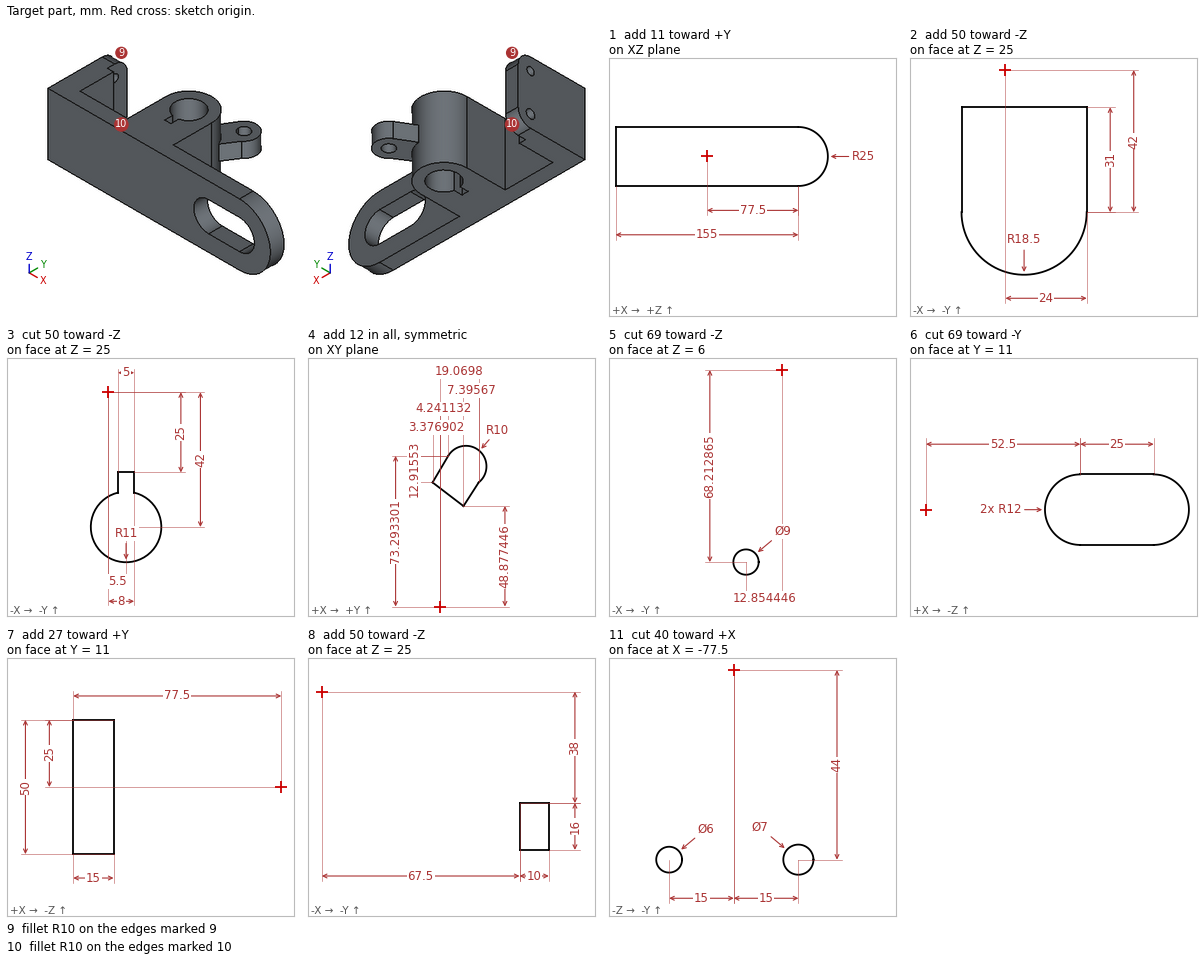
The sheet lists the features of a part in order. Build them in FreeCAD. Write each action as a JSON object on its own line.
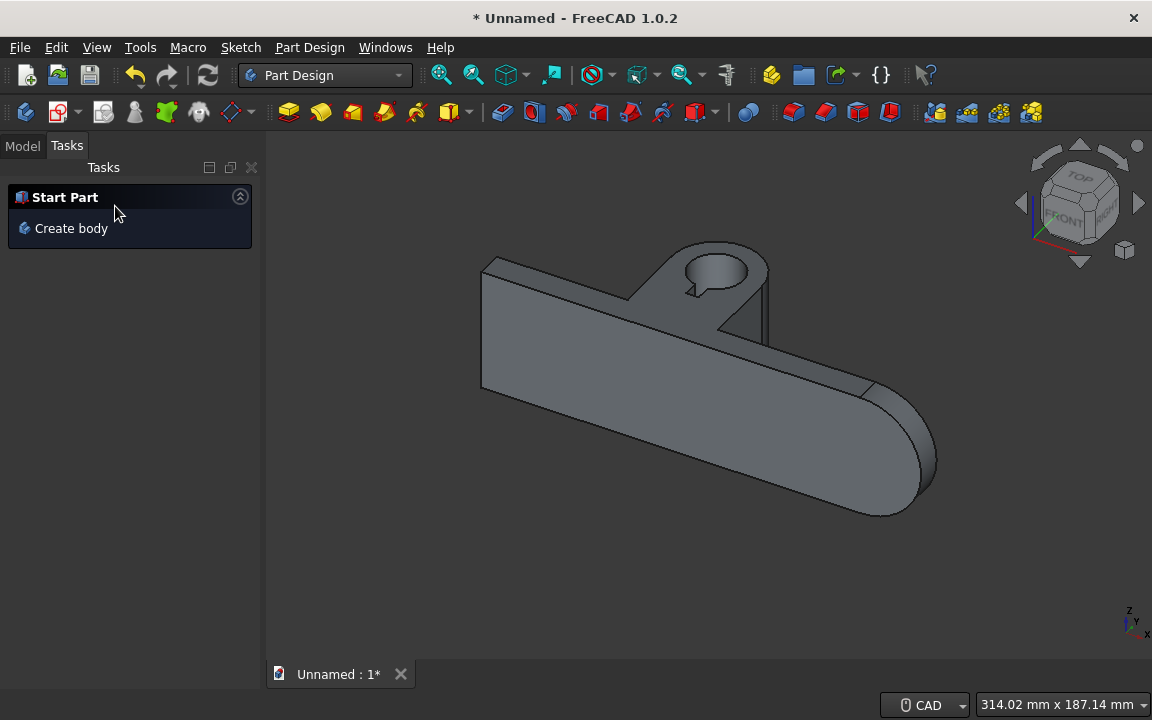
{"action": "left_click", "coordinate": [58, 112]}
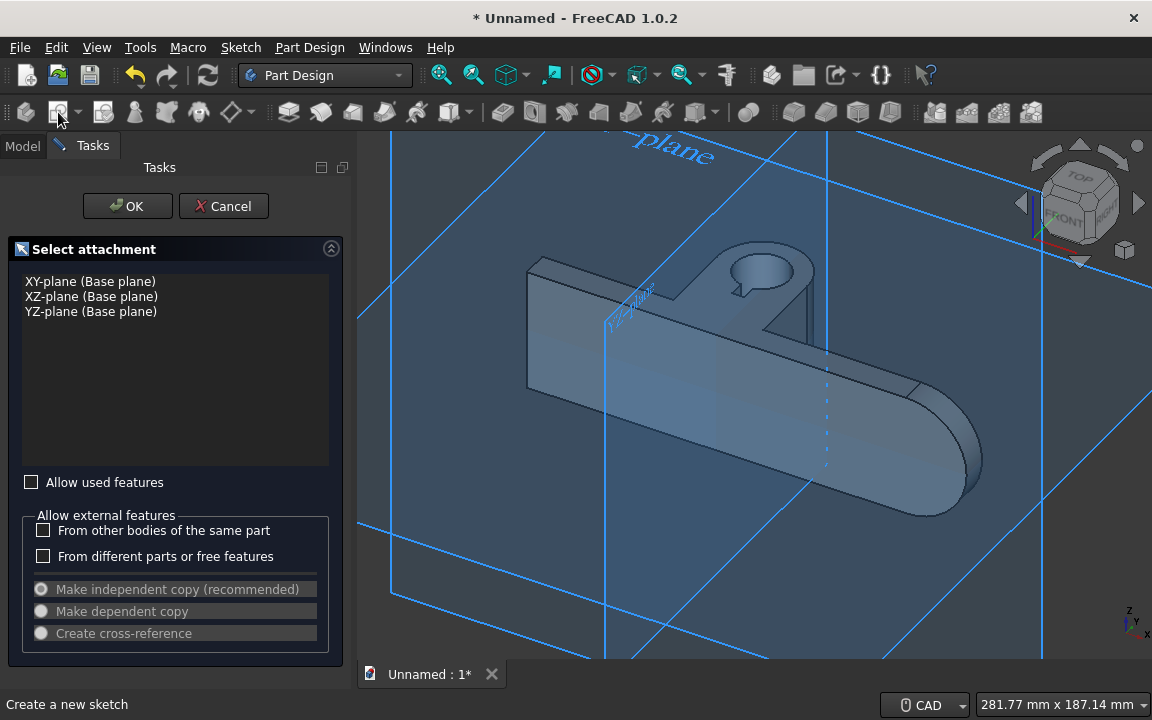
{"action": "left_click", "coordinate": [82, 282]}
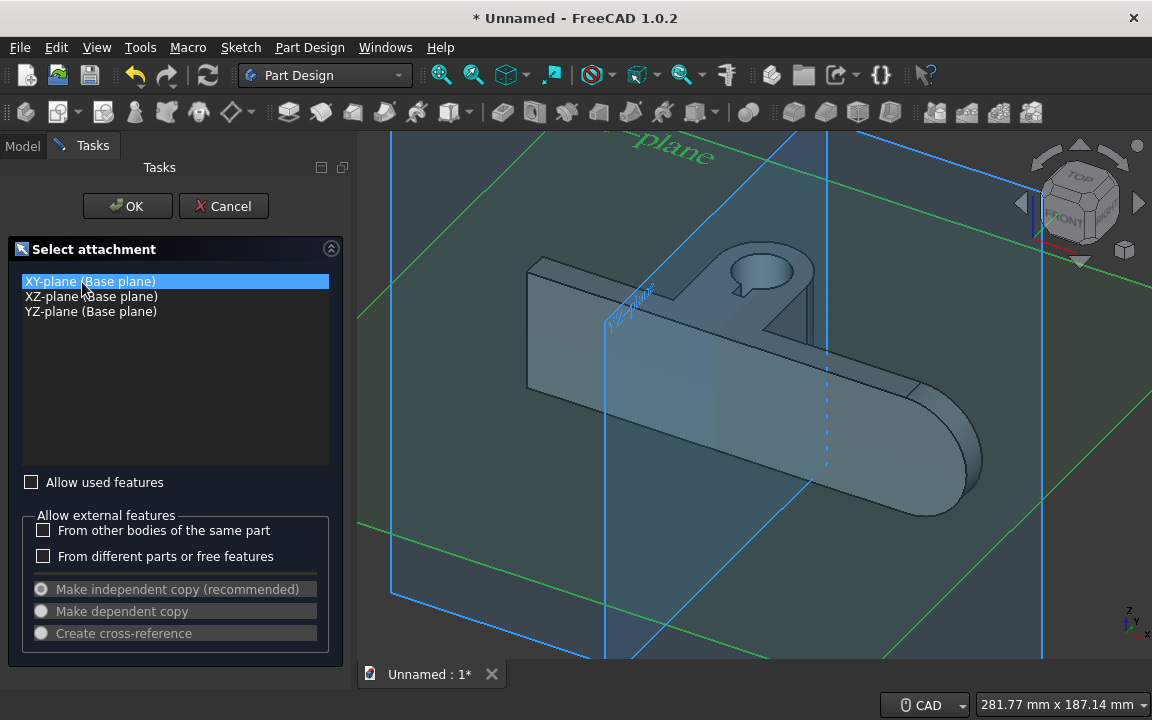
{"action": "left_click", "coordinate": [128, 206]}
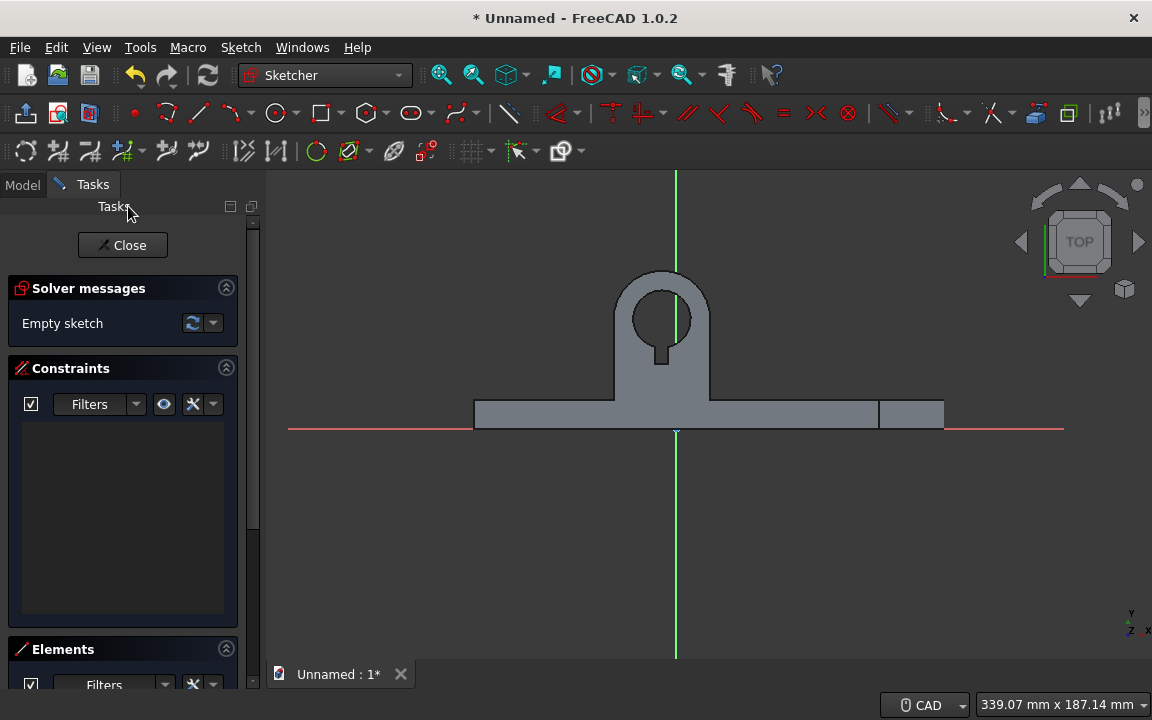
{"action": "left_click", "coordinate": [90, 114]}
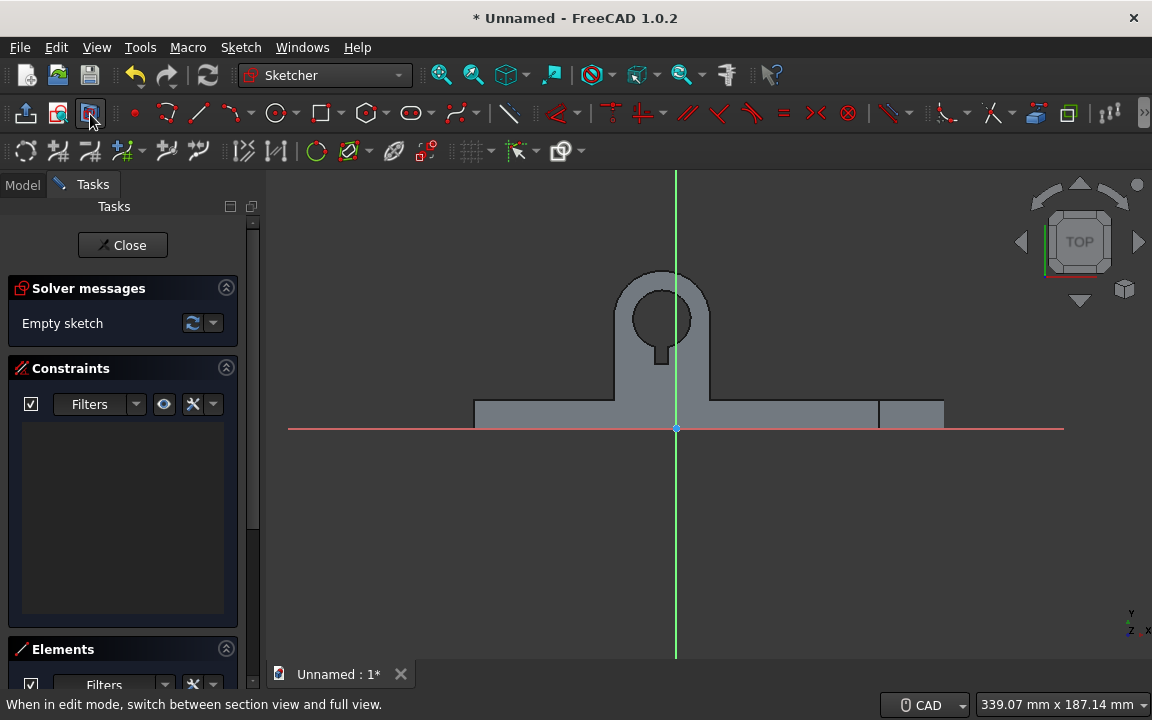
{"action": "scroll", "coordinate": [716, 217], "scroll_direction": "up", "scroll_amount": 7}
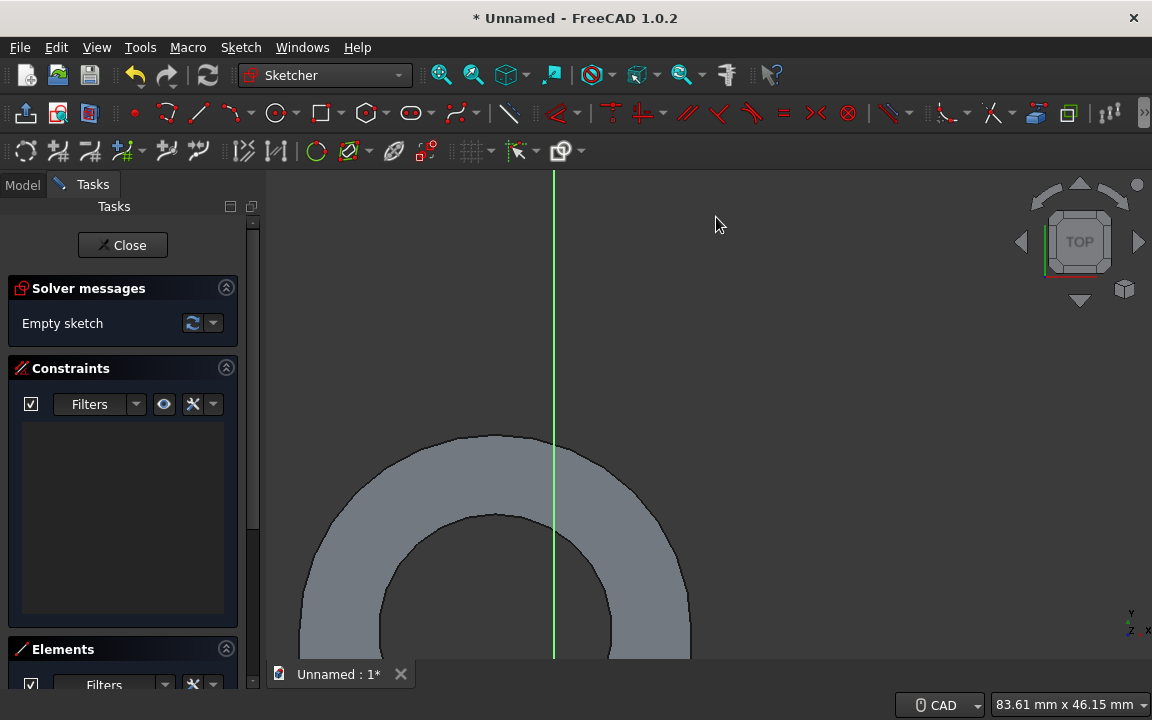
{"action": "left_click", "coordinate": [168, 114]}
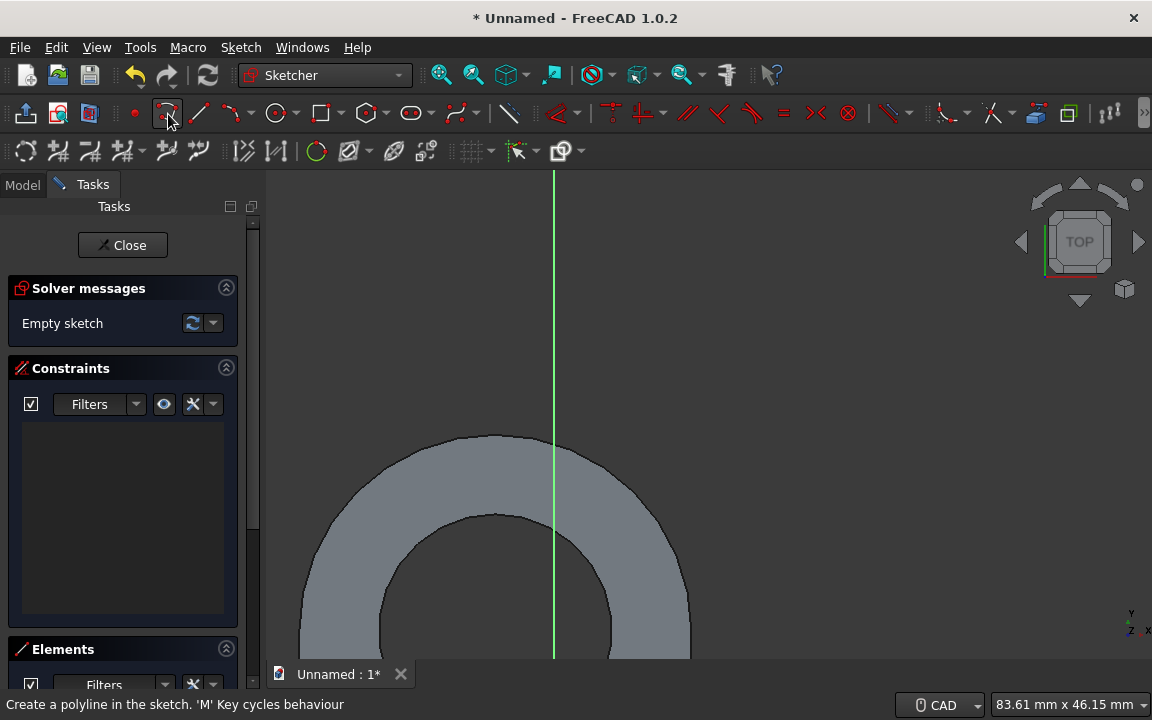
{"action": "left_click", "coordinate": [599, 299]}
{"action": "left_click", "coordinate": [518, 436]}
{"action": "left_click", "coordinate": [677, 558]}
{"action": "left_click", "coordinate": [756, 436]}
{"action": "right_click", "coordinate": [756, 436]}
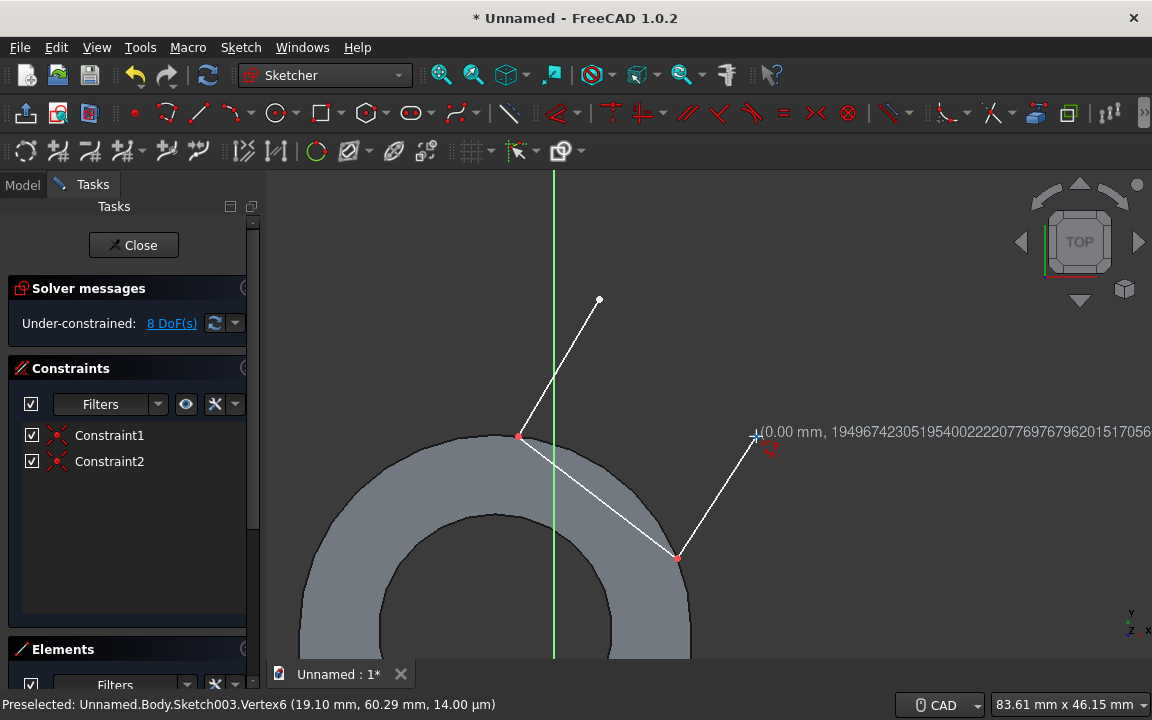
{"action": "left_click", "coordinate": [232, 114]}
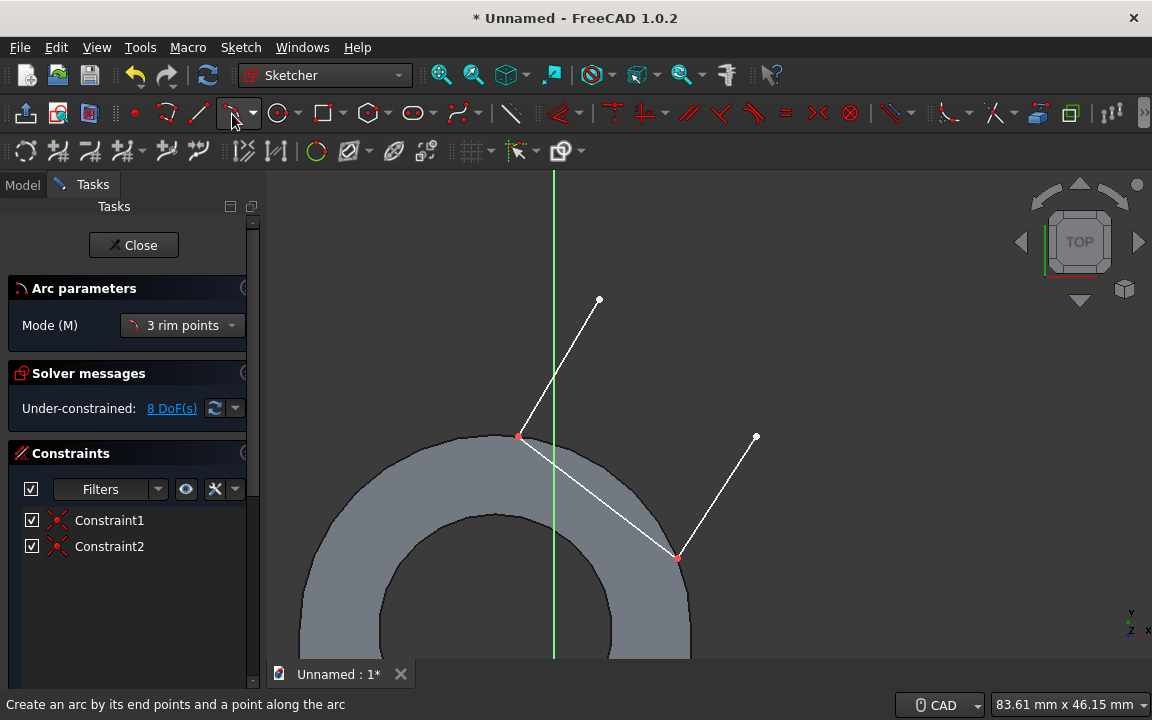
{"action": "left_click", "coordinate": [756, 437]}
{"action": "left_click", "coordinate": [599, 300]}
{"action": "left_click", "coordinate": [759, 273]}
{"action": "key", "text": "Escape"}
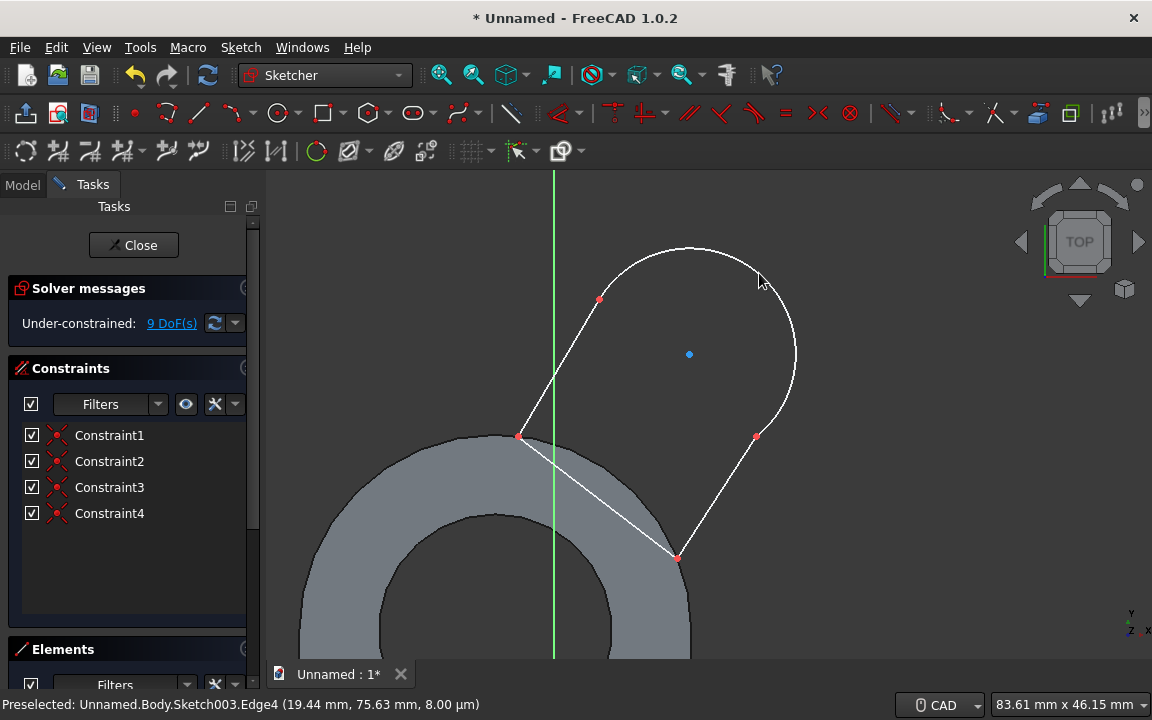
{"action": "left_click", "coordinate": [575, 341]}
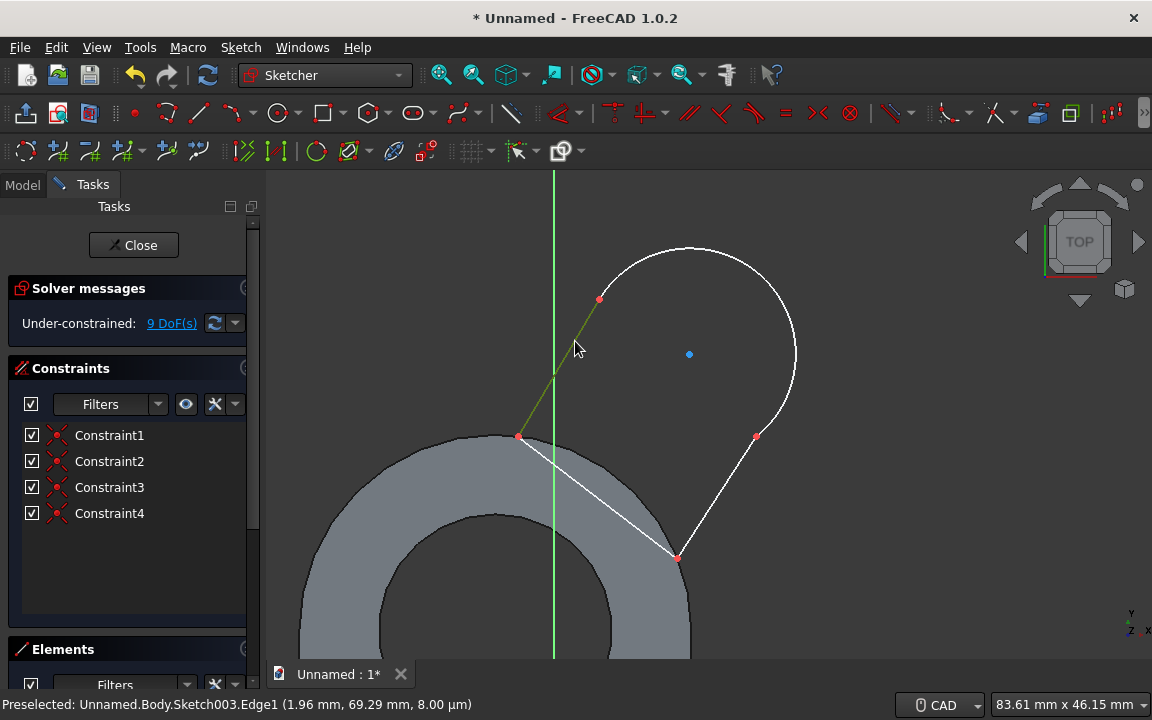
{"action": "left_click", "coordinate": [795, 338]}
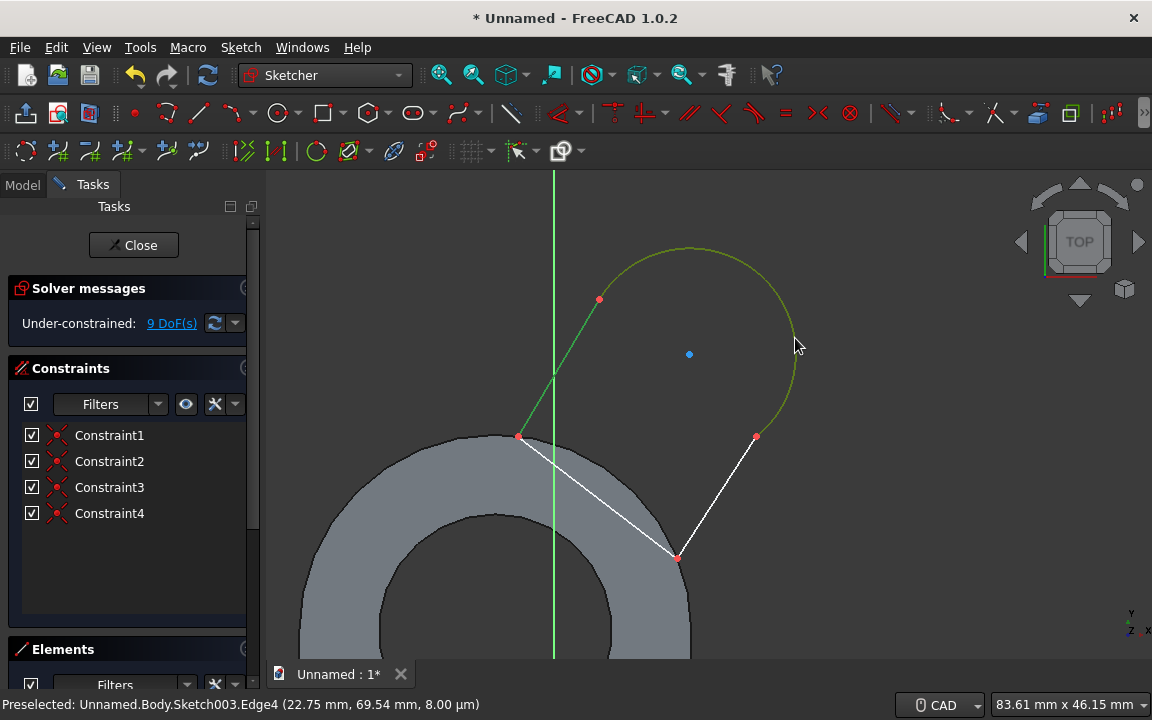
{"action": "left_click", "coordinate": [754, 114]}